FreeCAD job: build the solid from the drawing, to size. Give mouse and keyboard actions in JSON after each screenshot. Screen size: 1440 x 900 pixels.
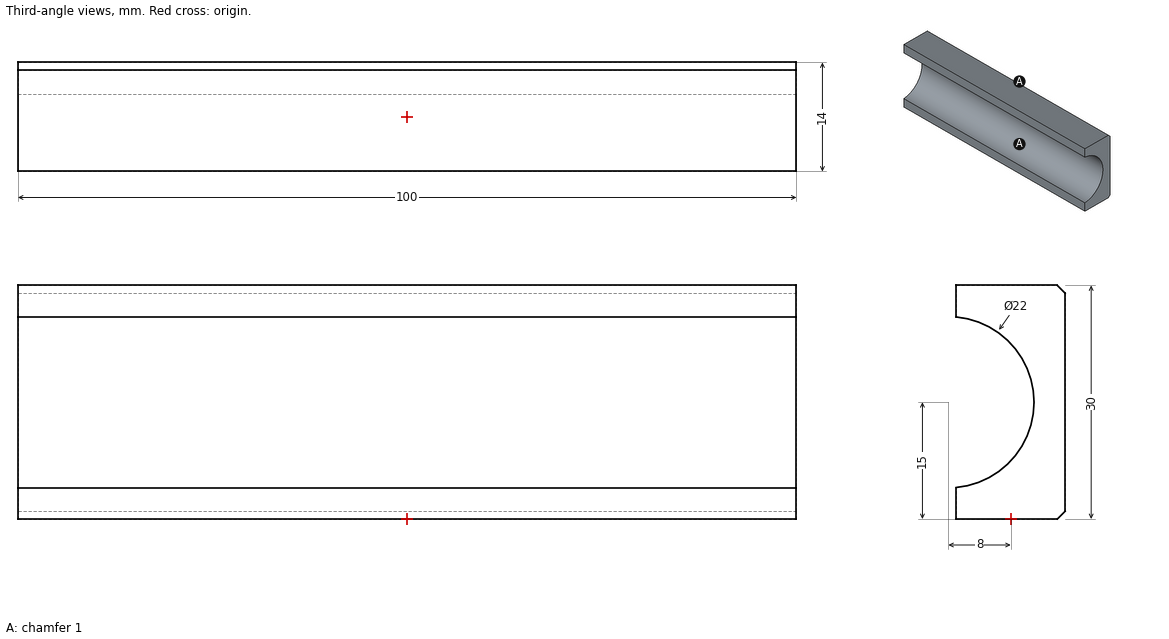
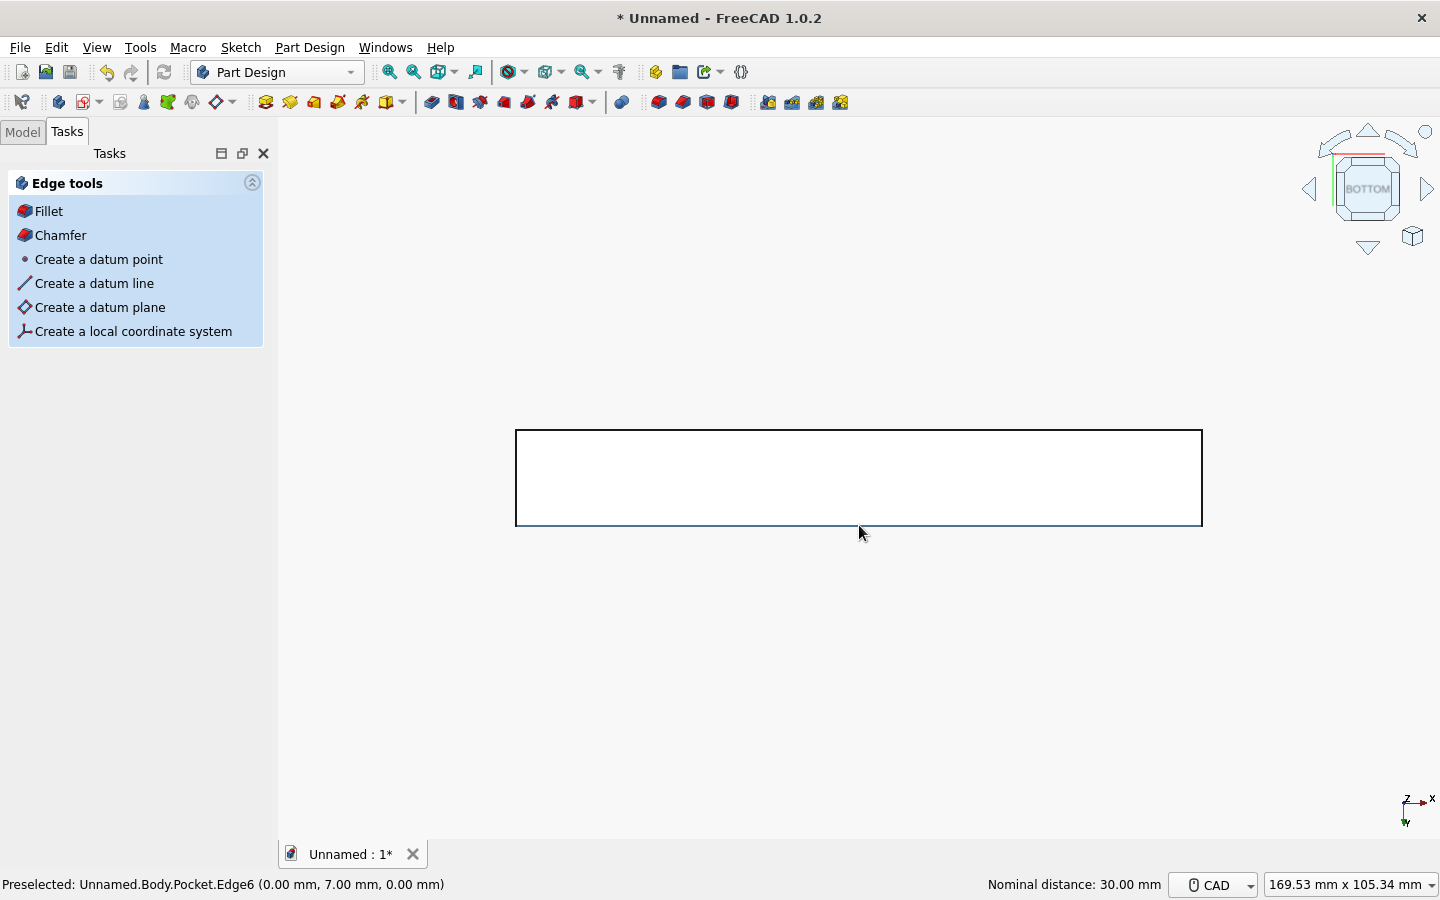
{"action": "left_click", "coordinate": [684, 102]}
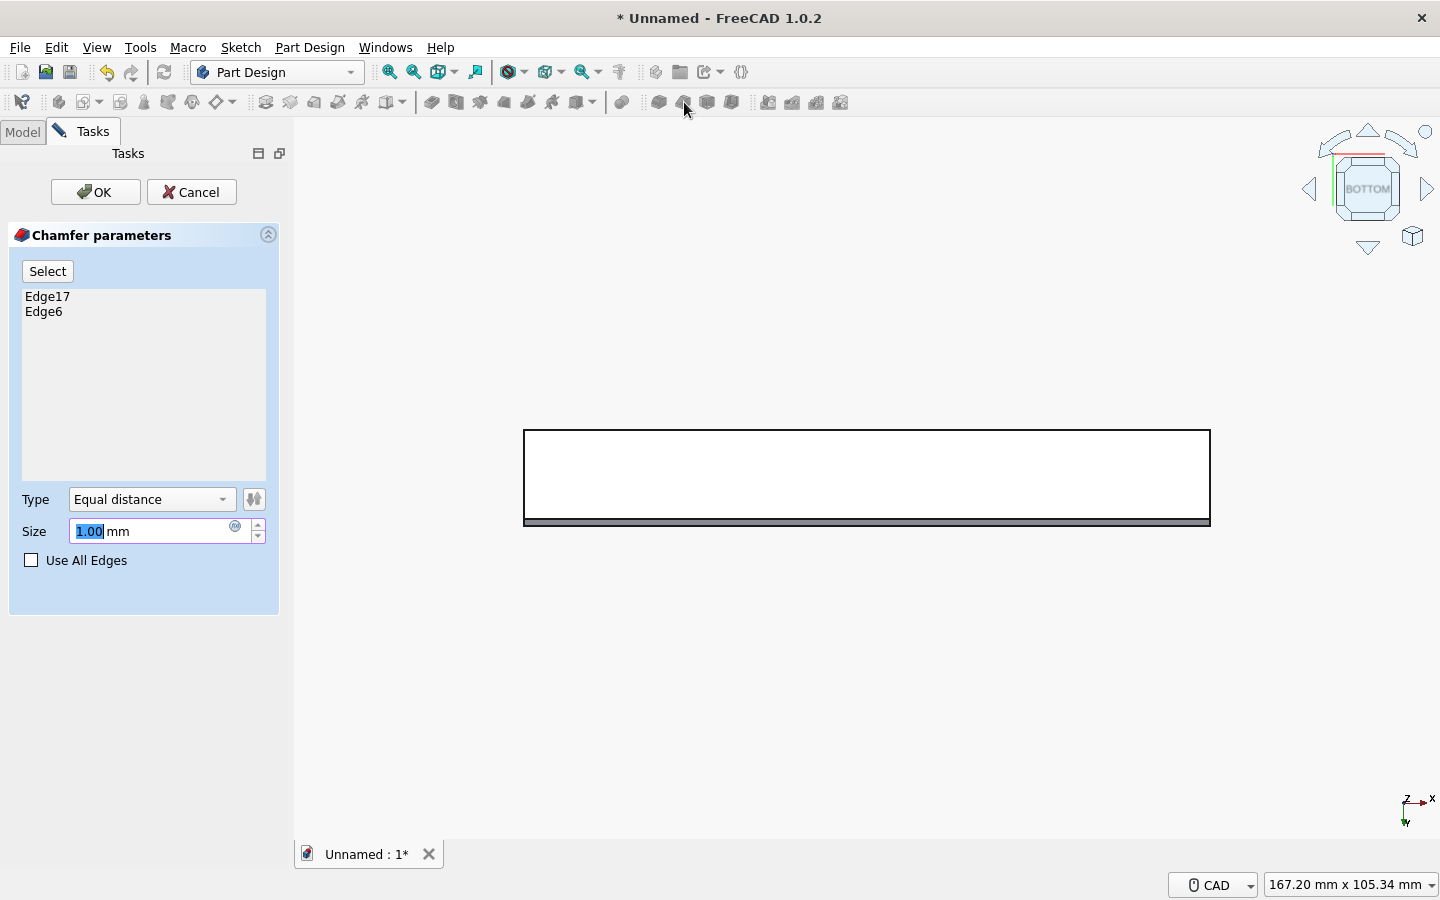
{"action": "type", "text": "1"}
{"action": "key", "text": "Tab"}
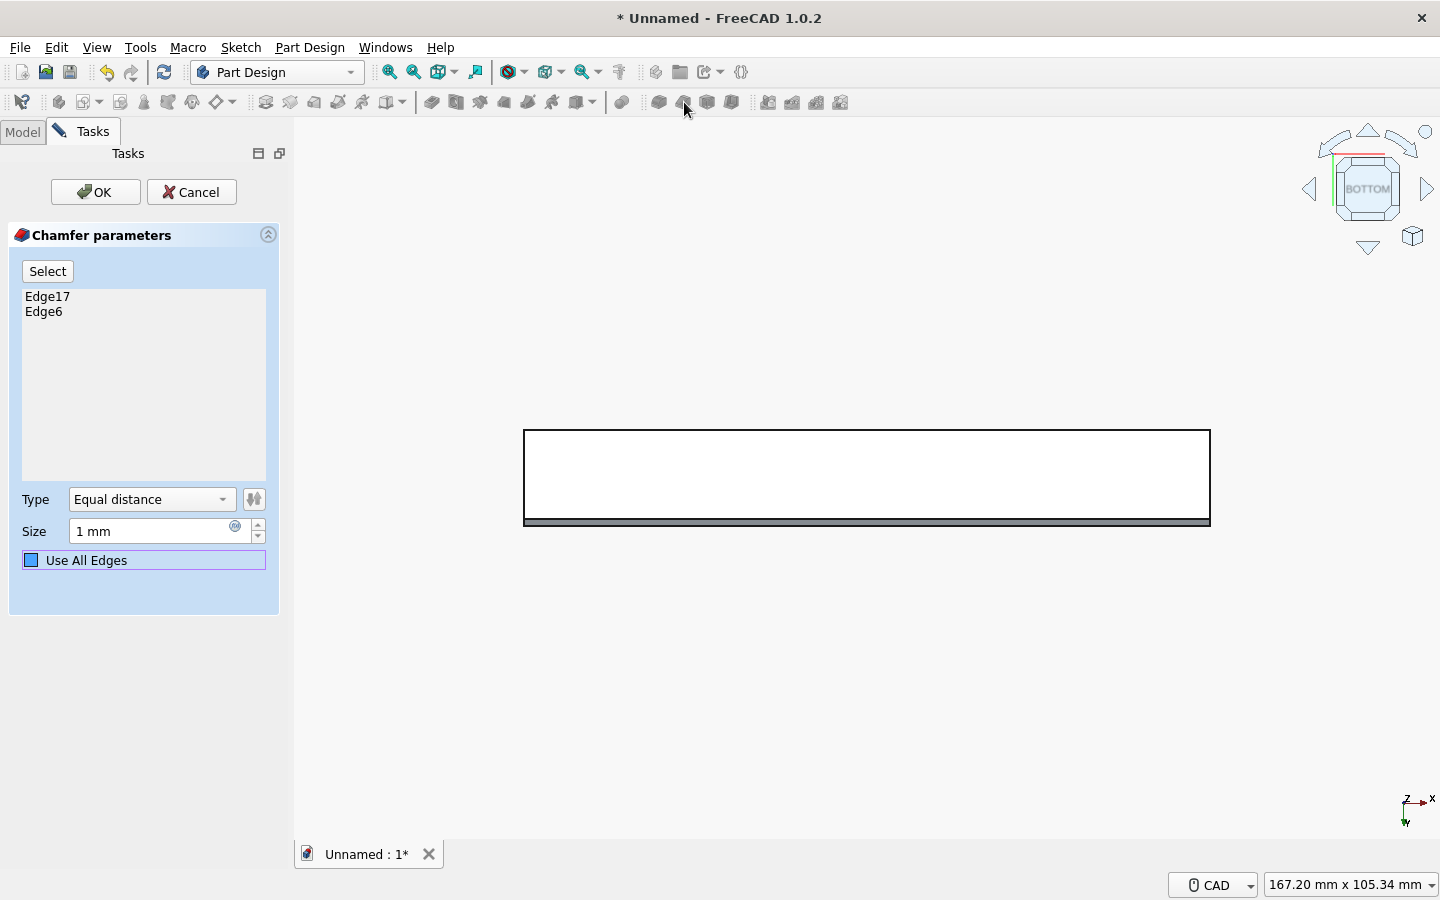
{"action": "left_click", "coordinate": [96, 192]}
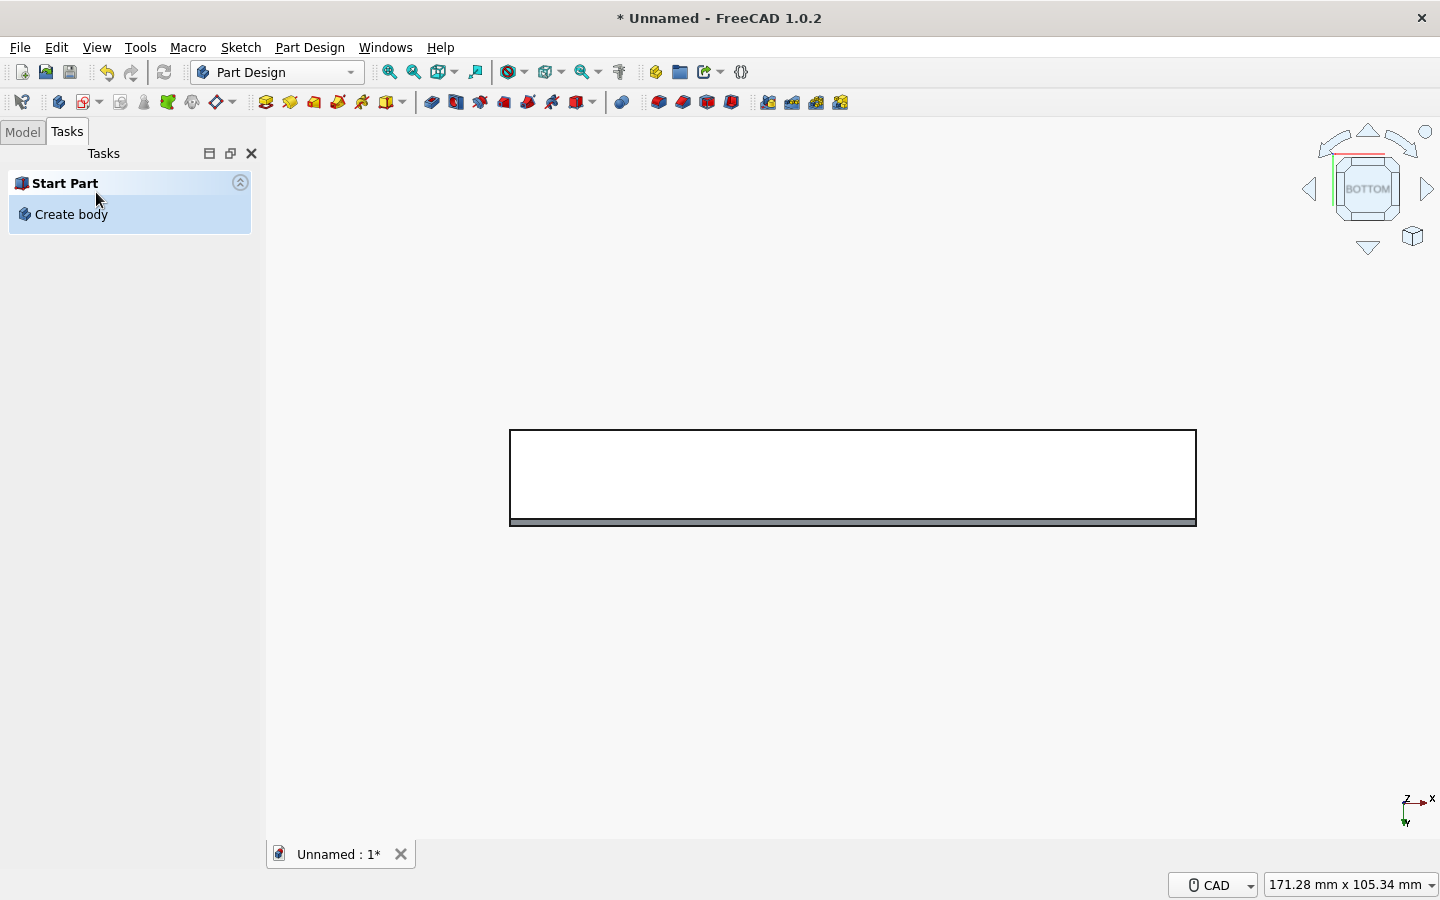
{"action": "key", "text": "0"}